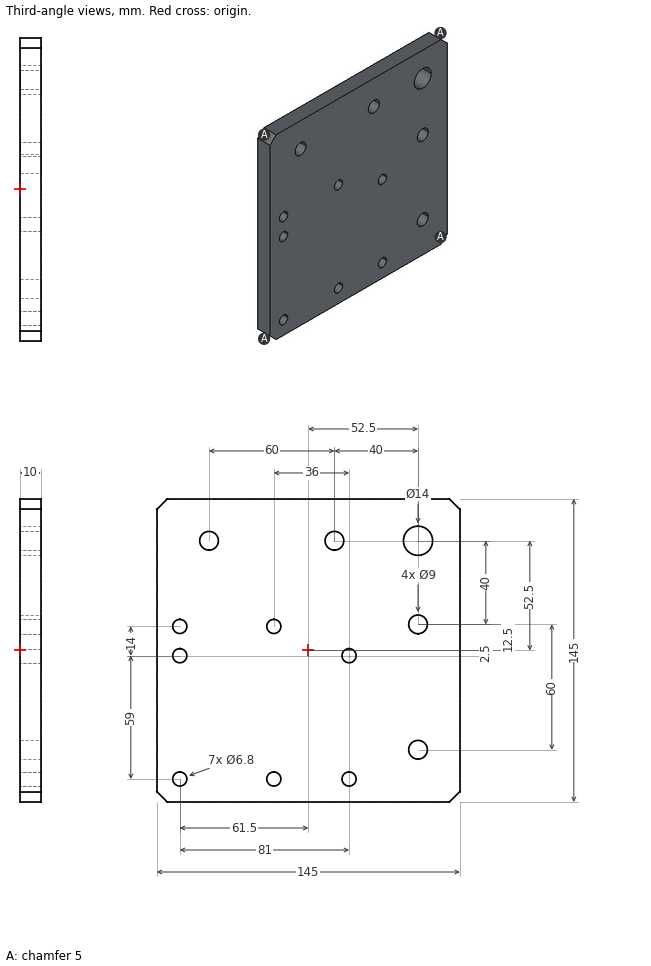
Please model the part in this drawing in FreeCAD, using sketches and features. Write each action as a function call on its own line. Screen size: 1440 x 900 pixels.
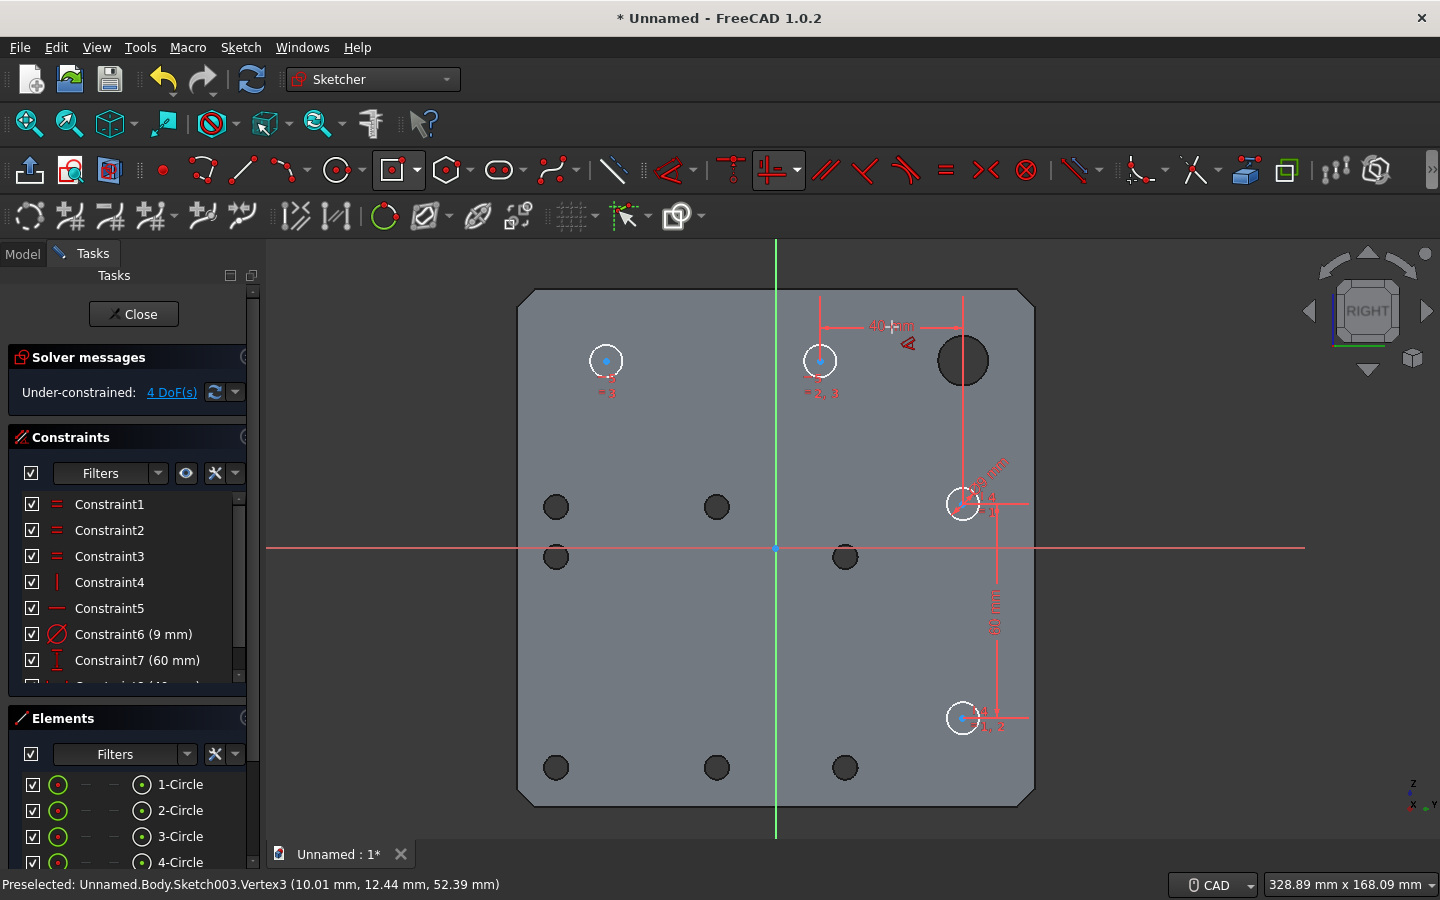
click(963, 504)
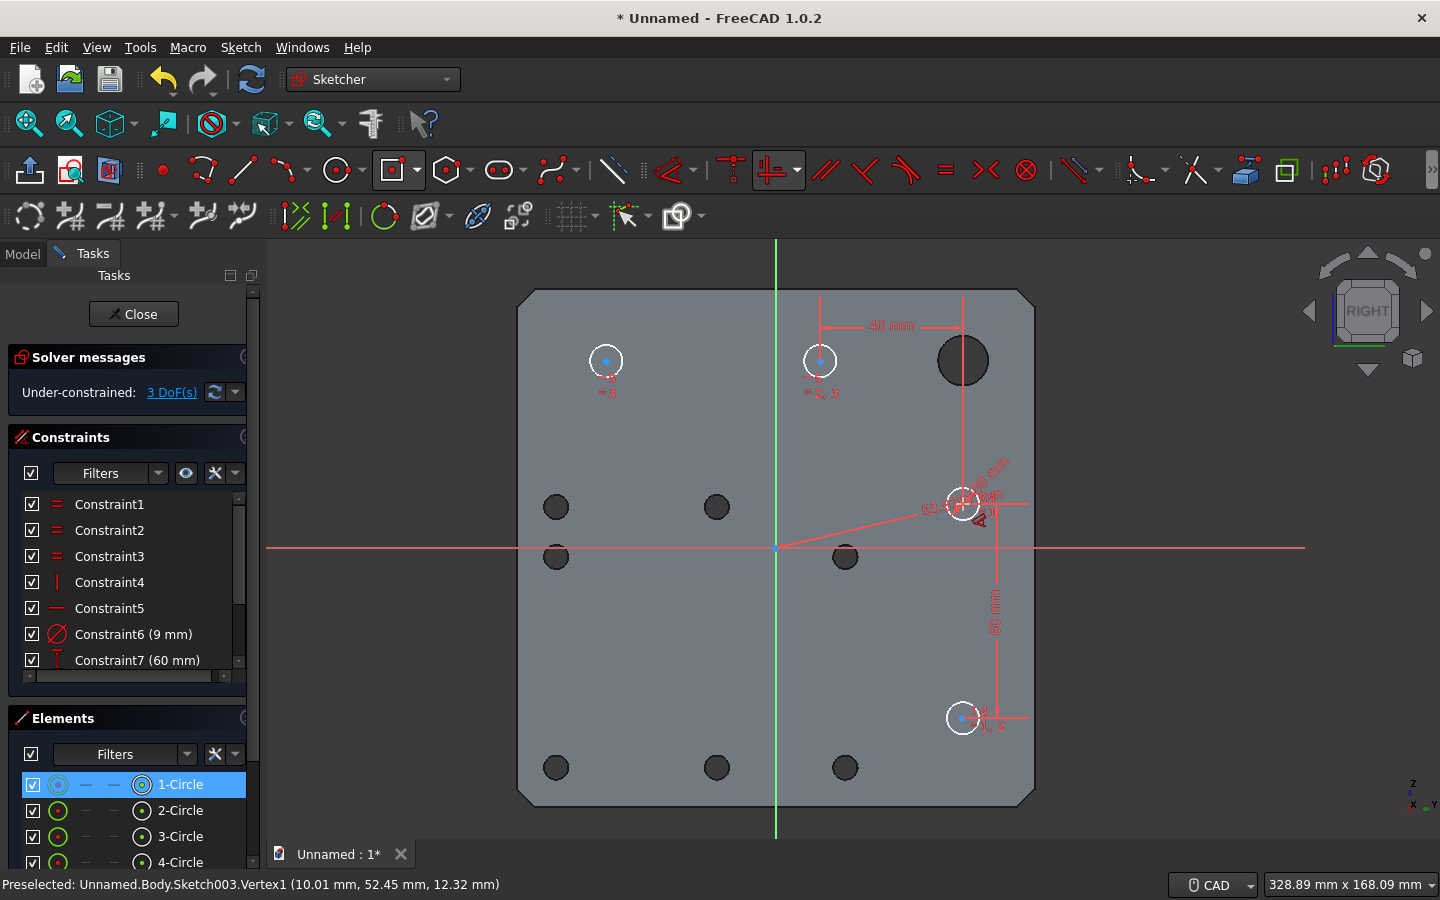
click(820, 361)
click(997, 433)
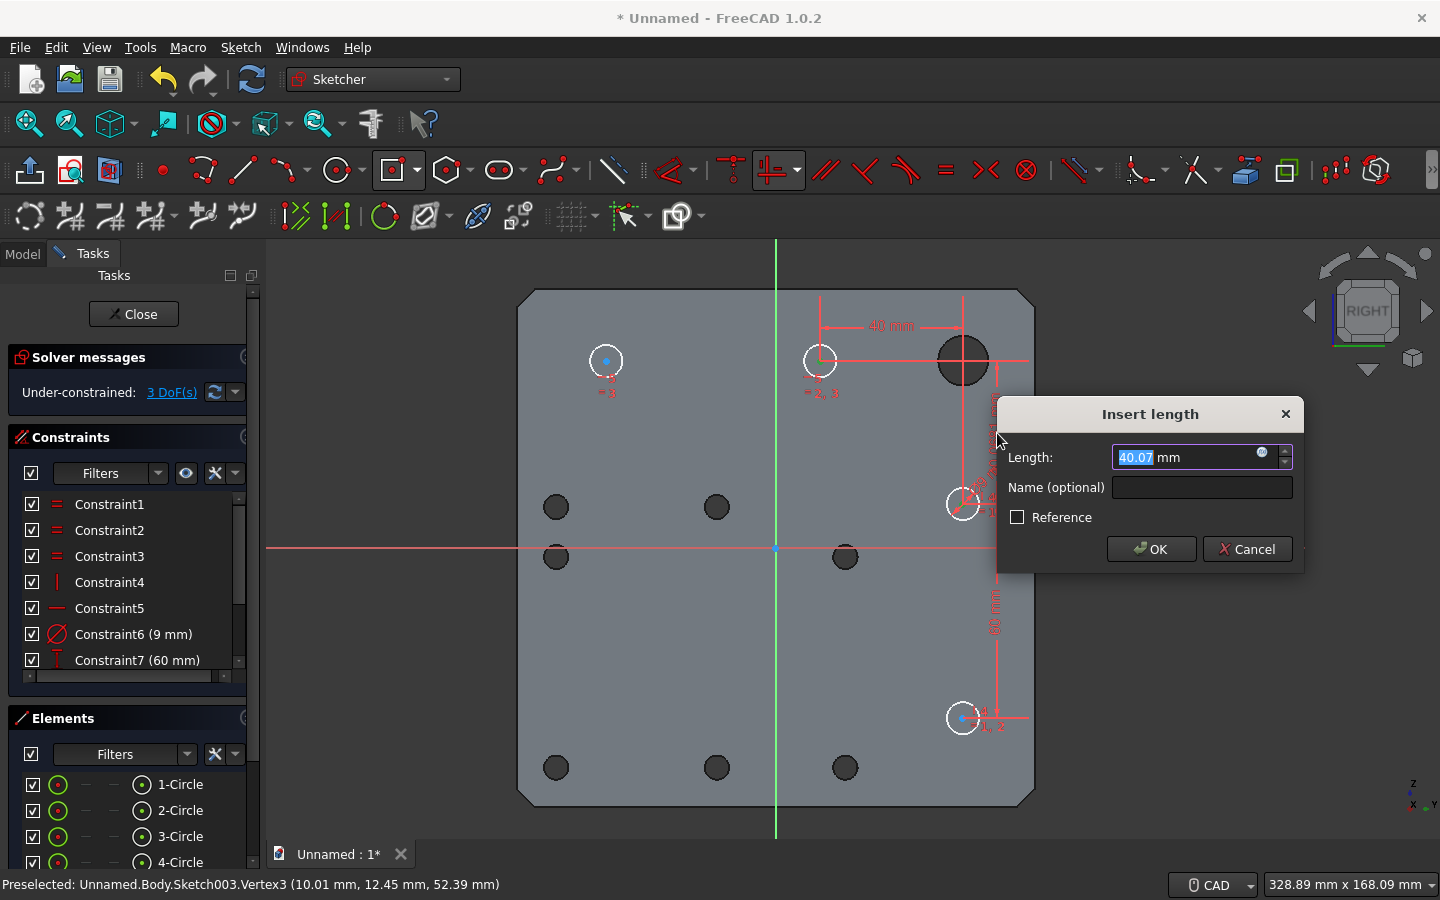
text(40)
key(Return)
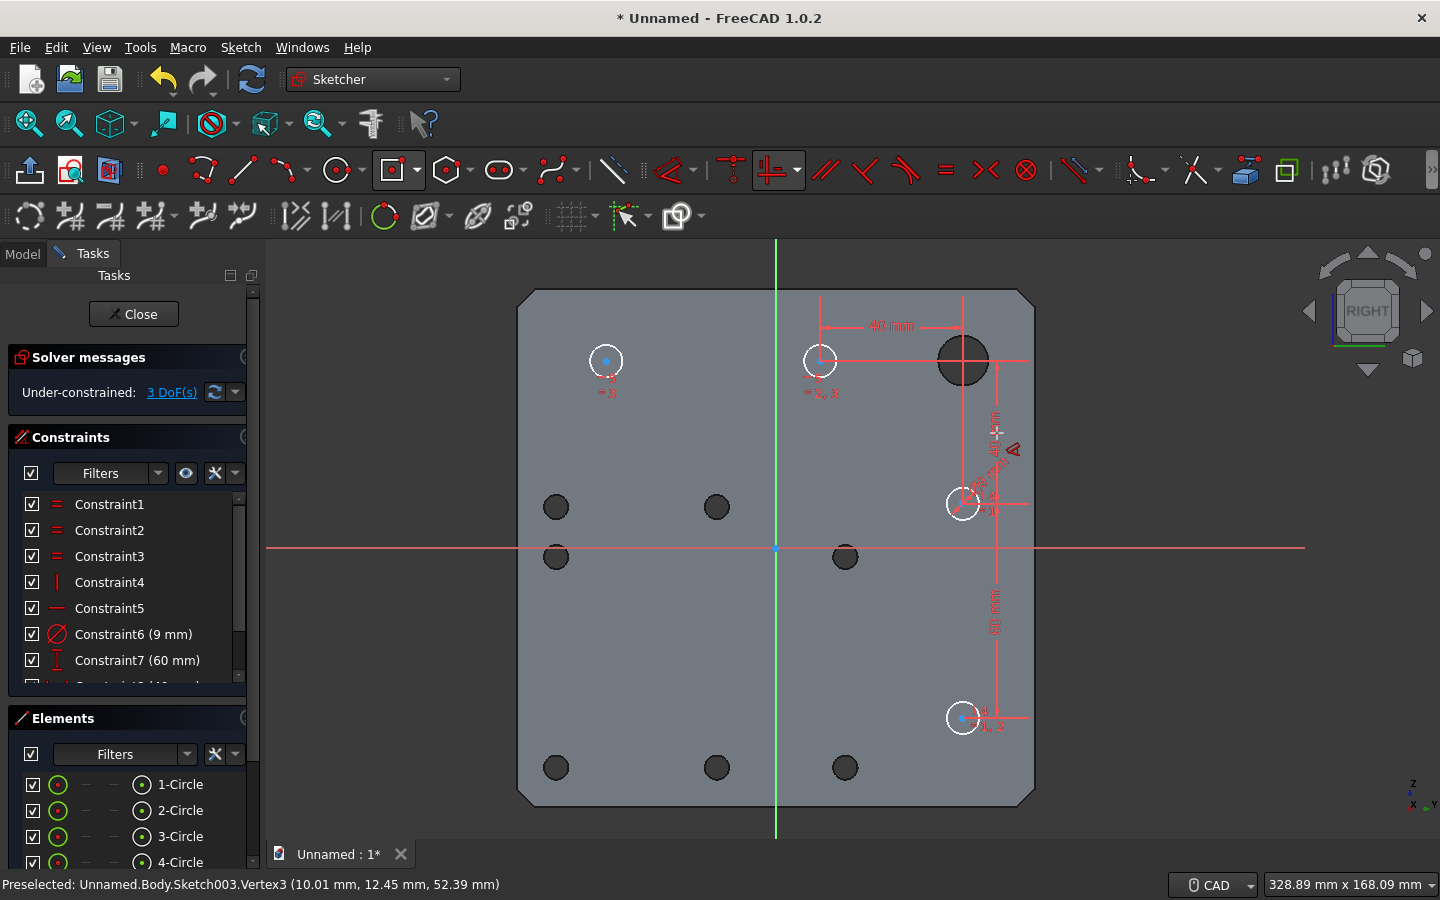
click(820, 361)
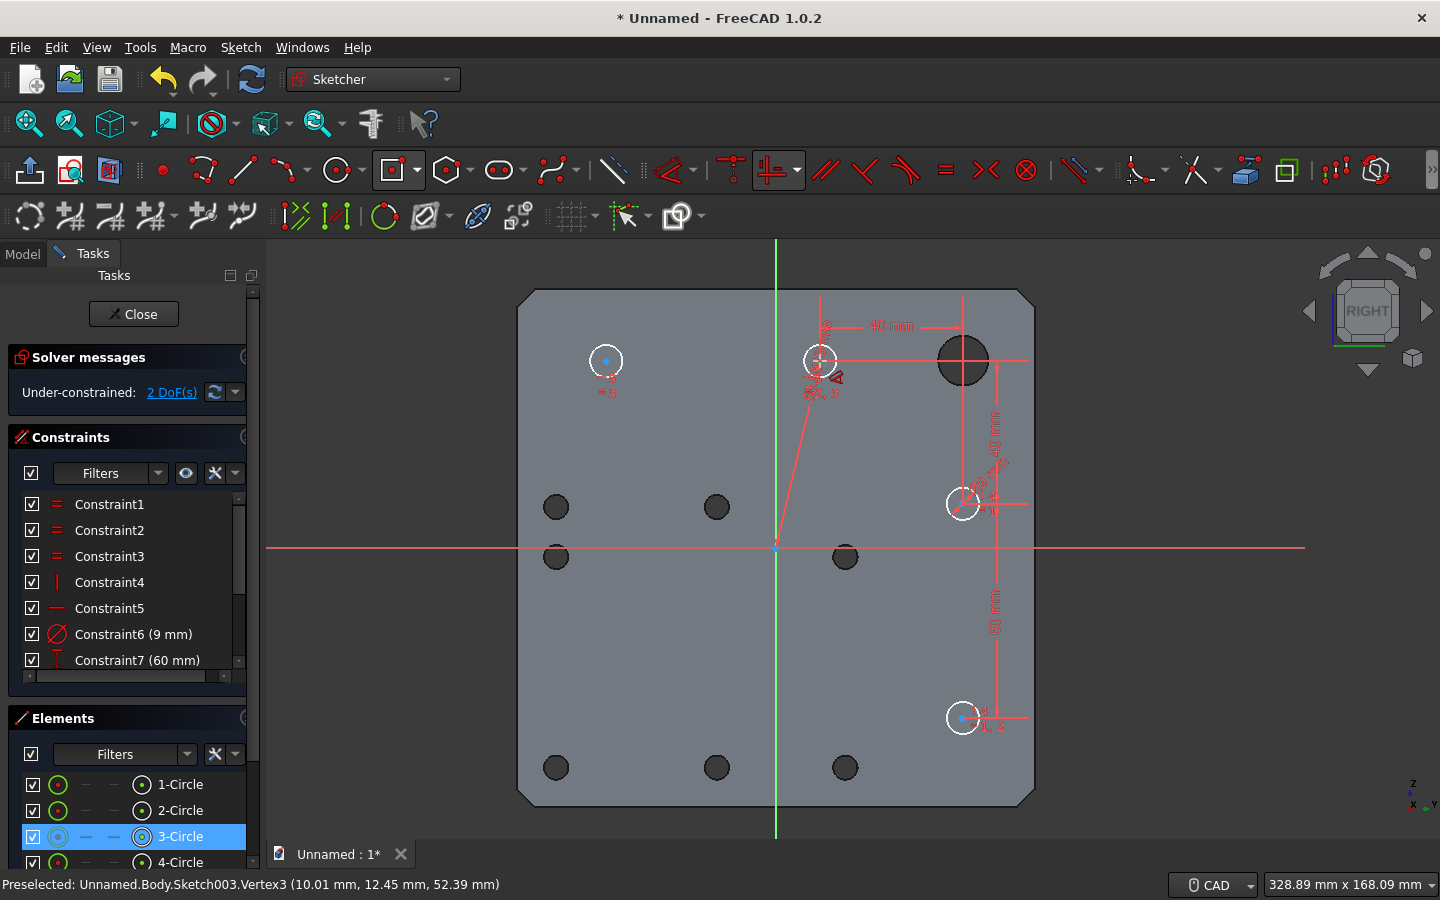
click(606, 361)
click(713, 327)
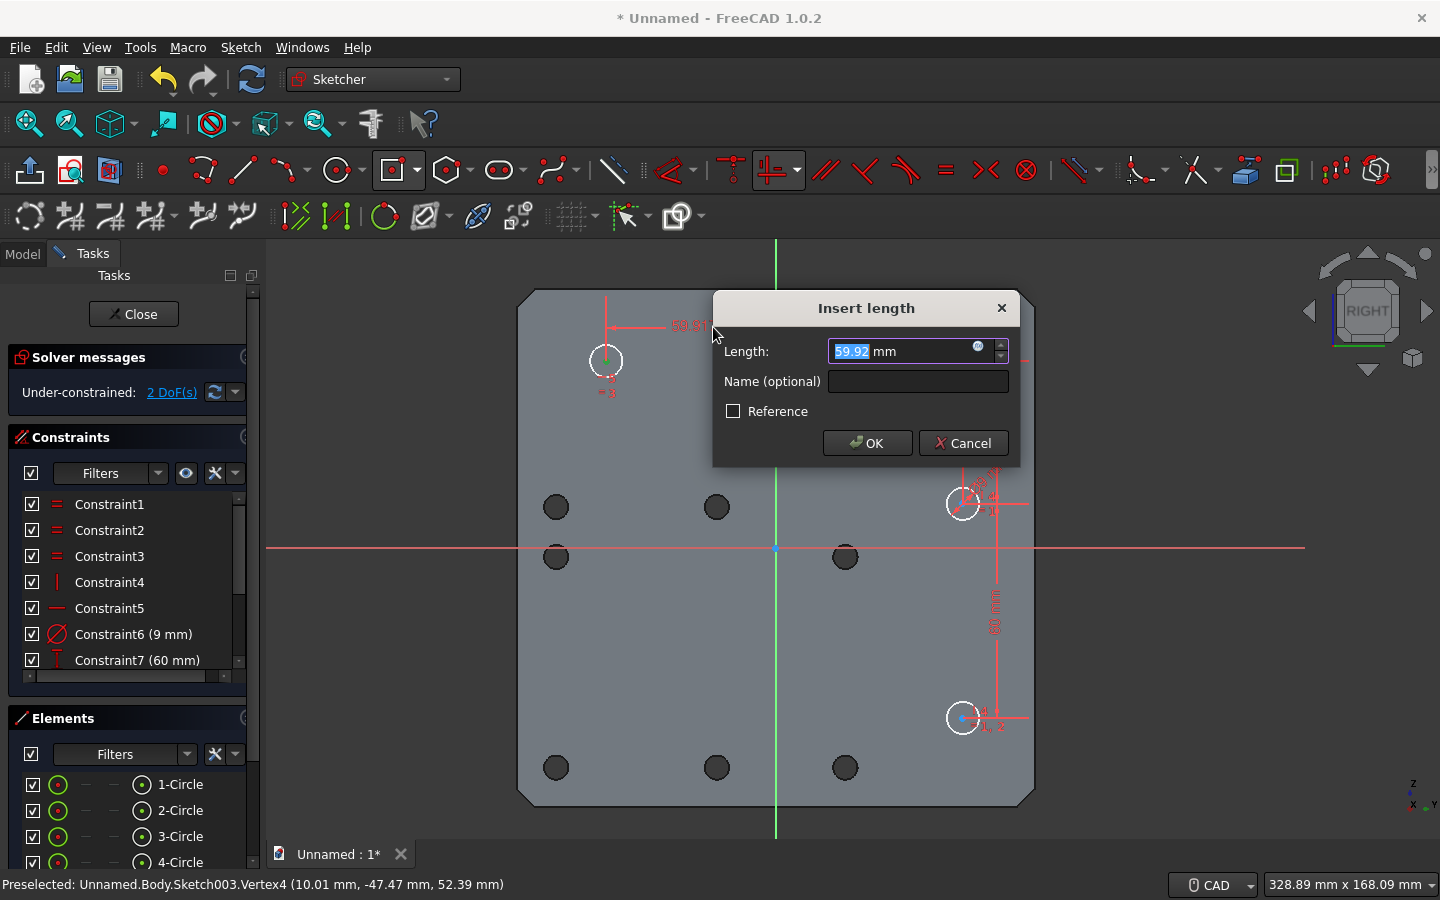
text(60)
key(Return)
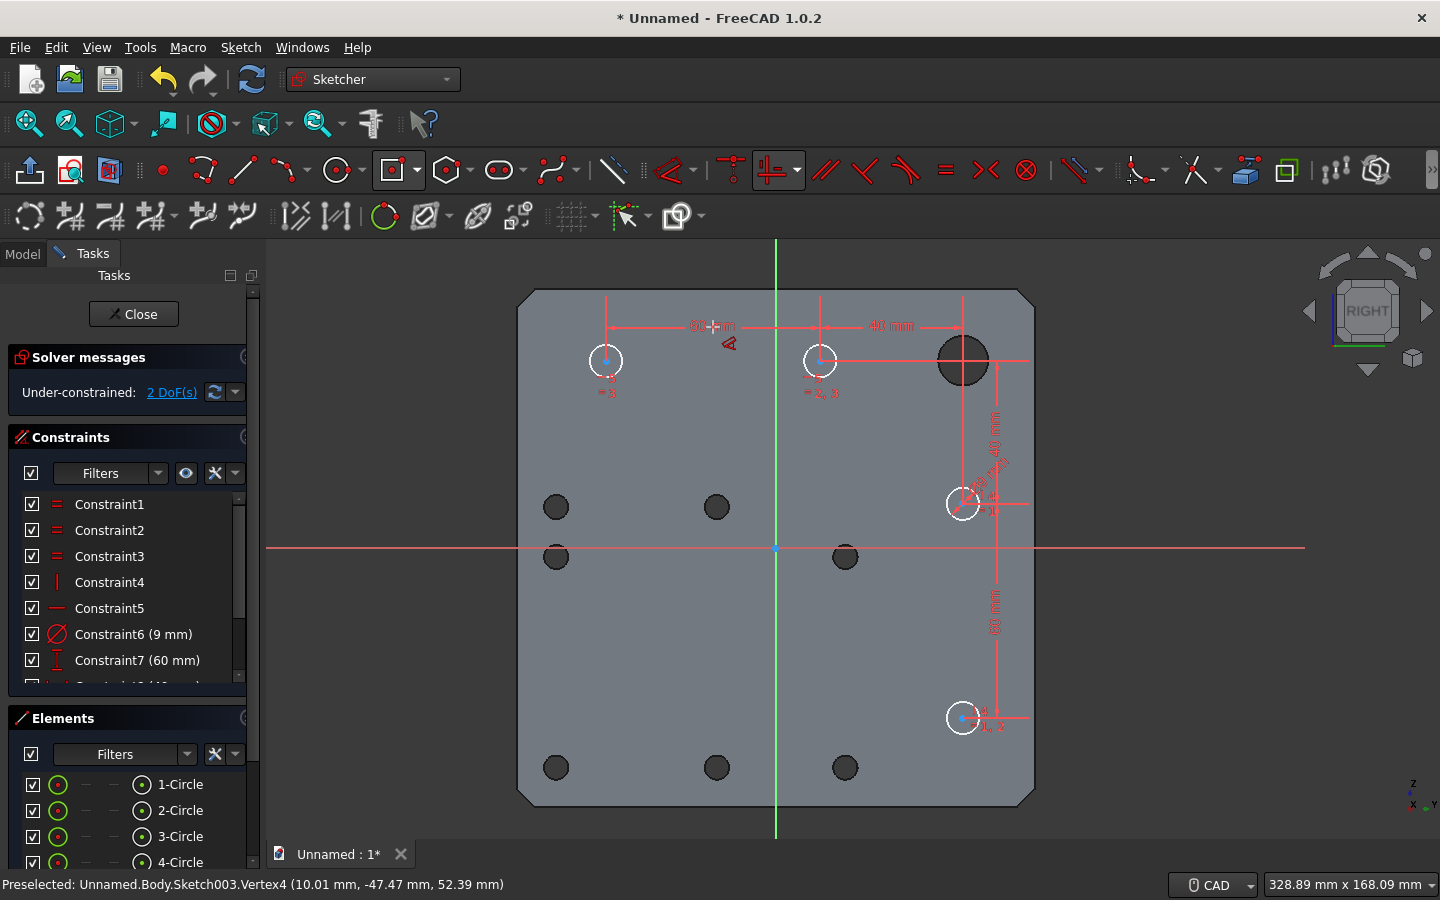
click(963, 504)
click(869, 470)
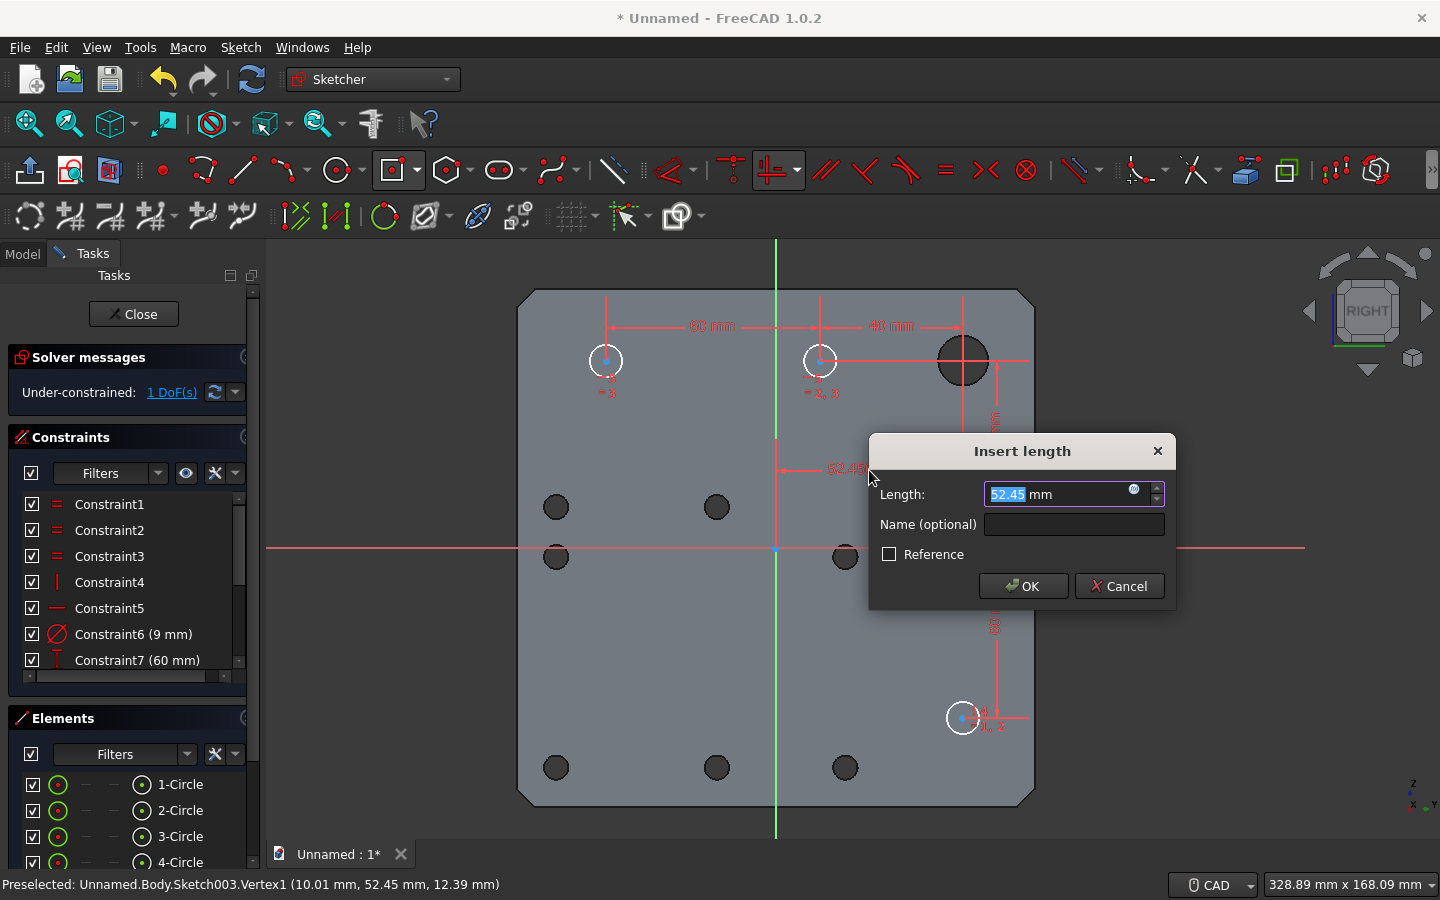
text(52.5)
key(Return)